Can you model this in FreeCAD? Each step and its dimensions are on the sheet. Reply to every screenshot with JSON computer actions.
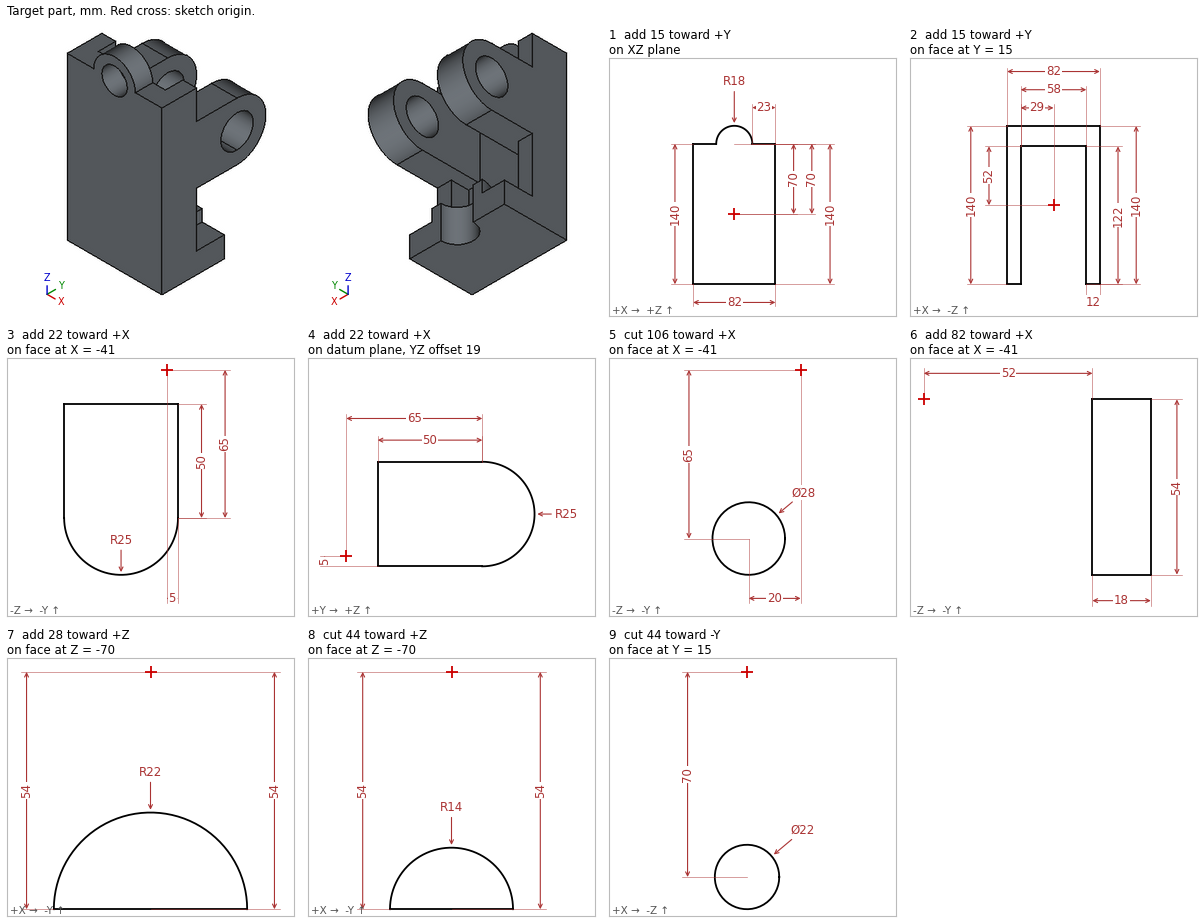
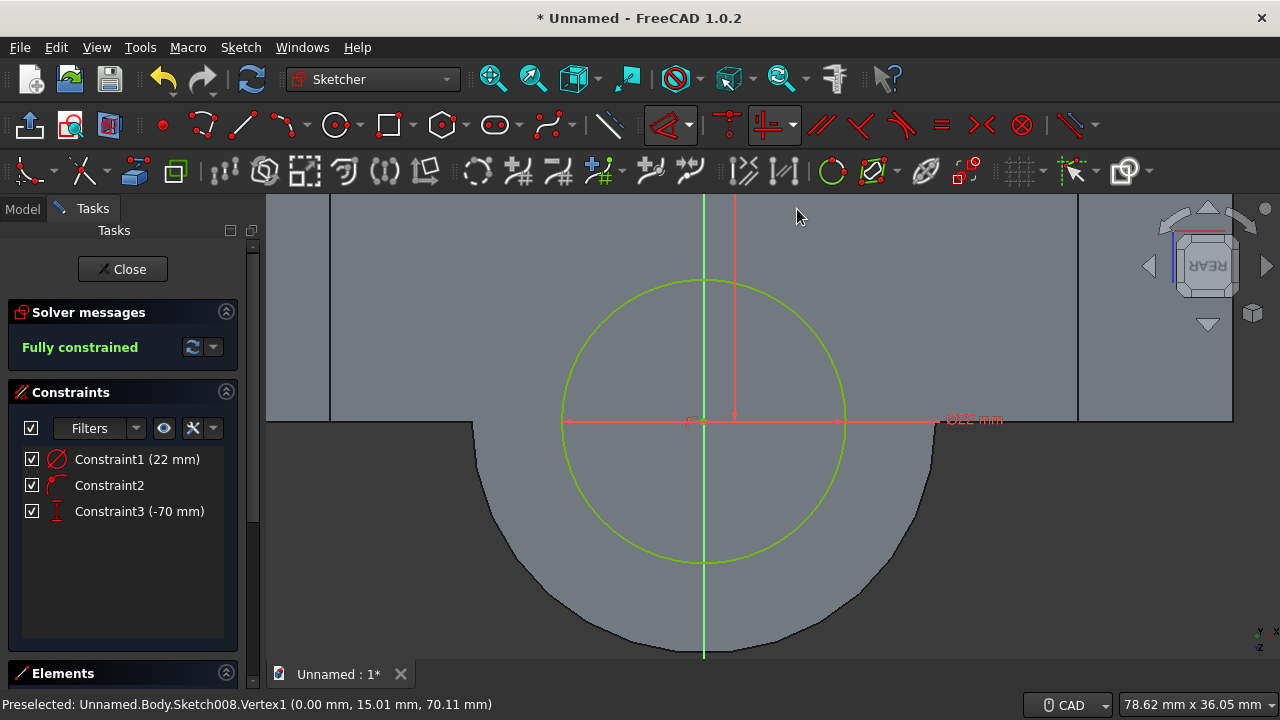
{"action": "left_click", "coordinate": [123, 269]}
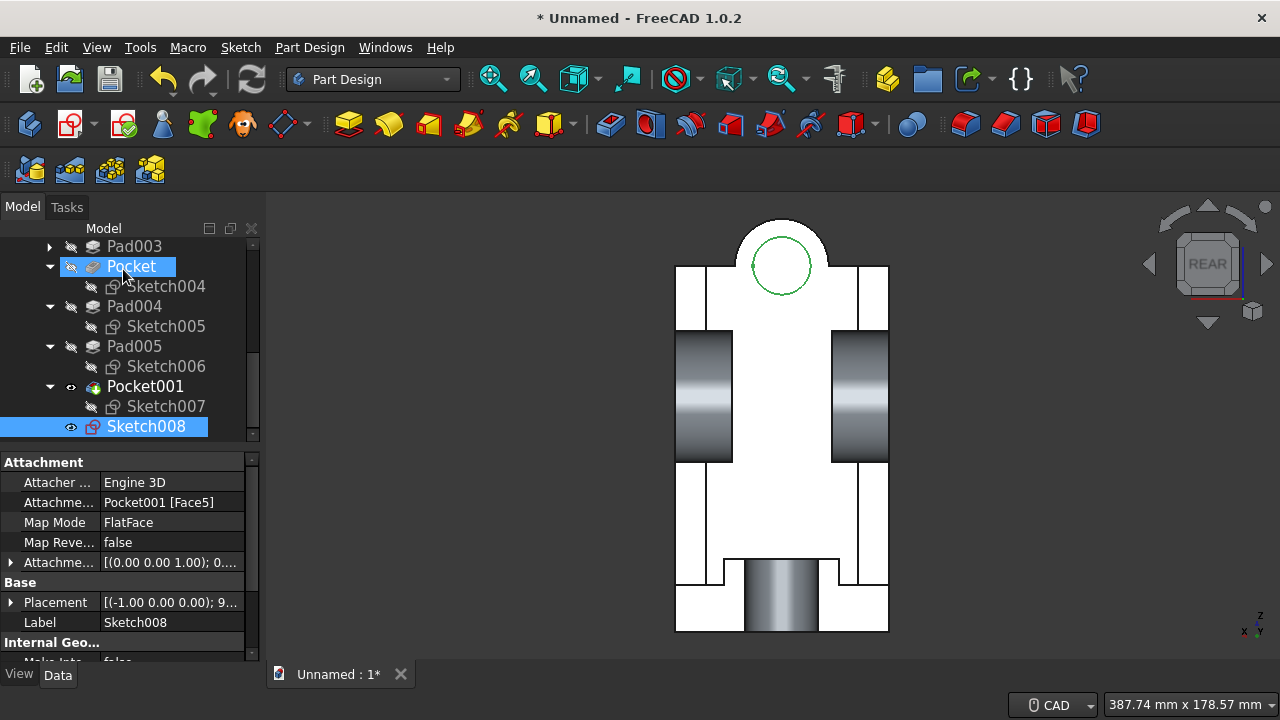
{"action": "left_click", "coordinate": [612, 124]}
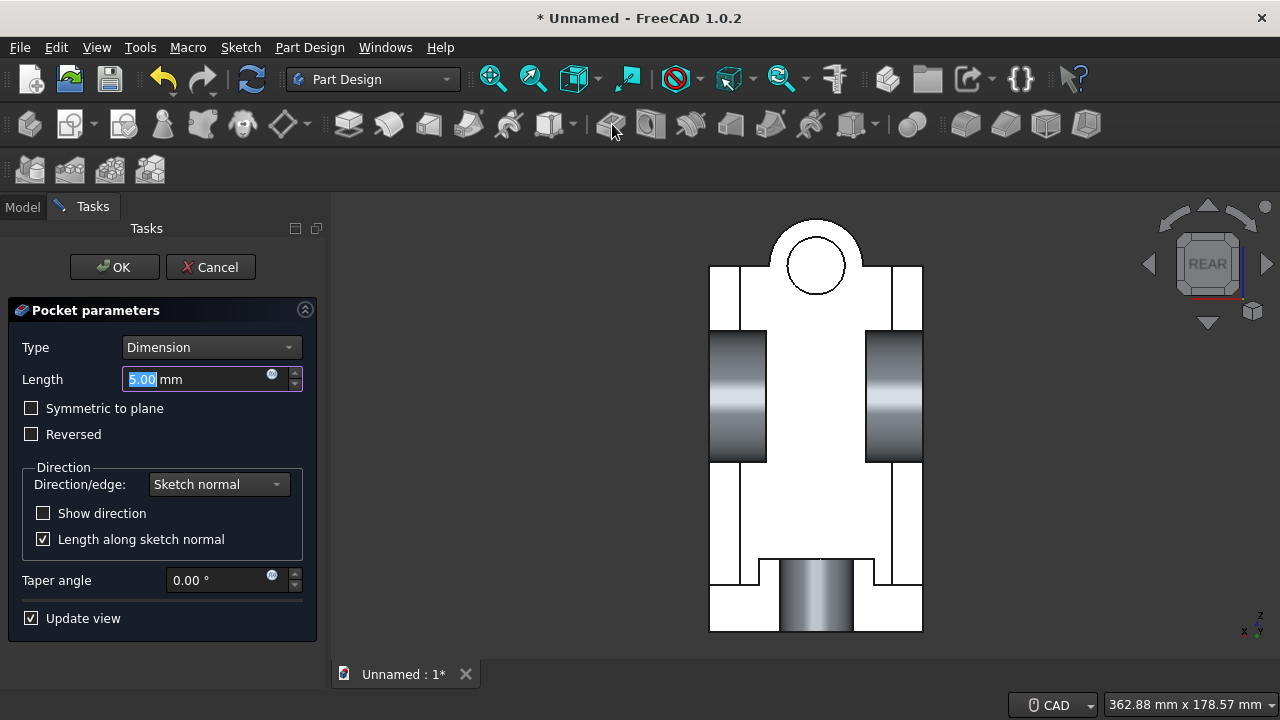
{"action": "type", "text": "44"}
{"action": "key", "text": "Tab"}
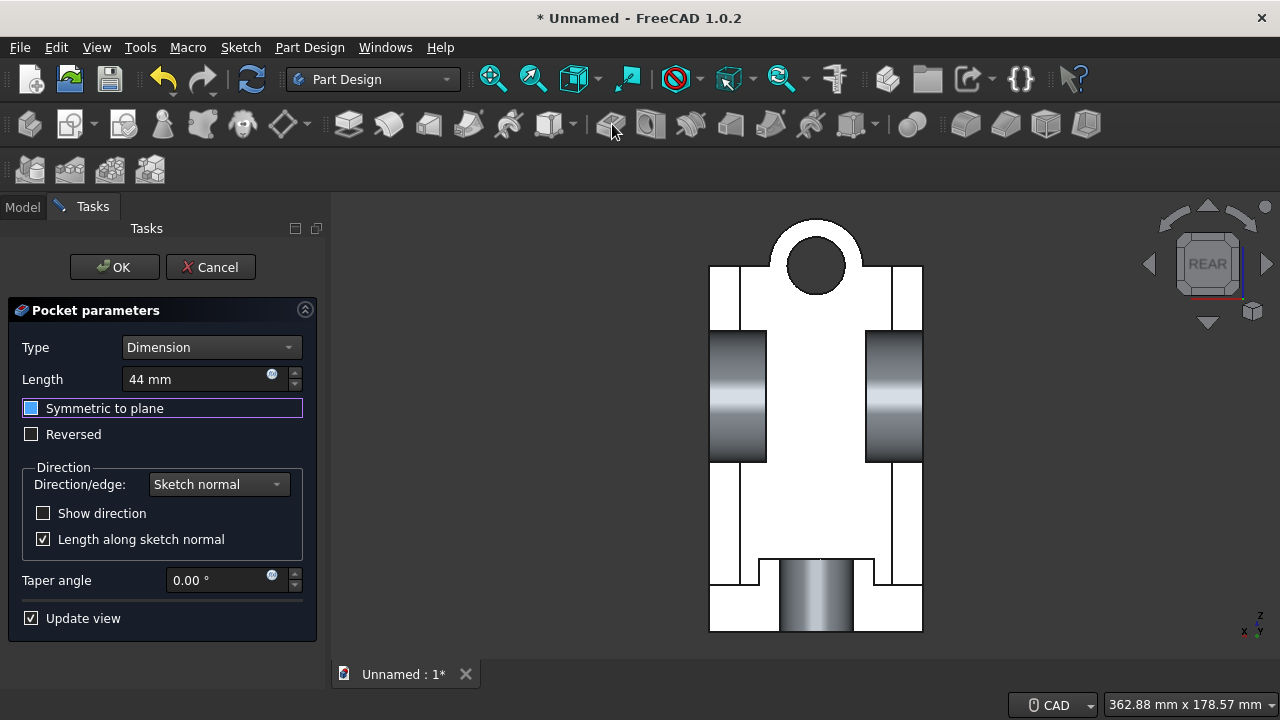
{"action": "left_click", "coordinate": [115, 267]}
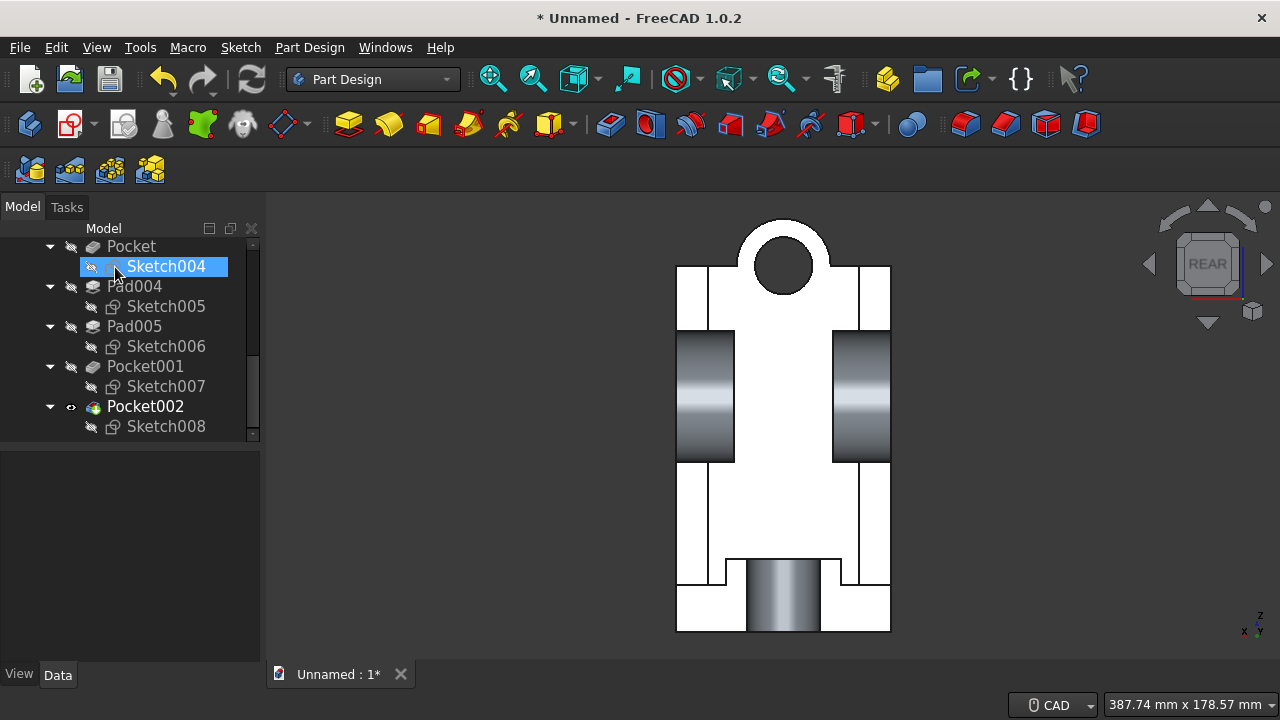
{"action": "key", "text": "0"}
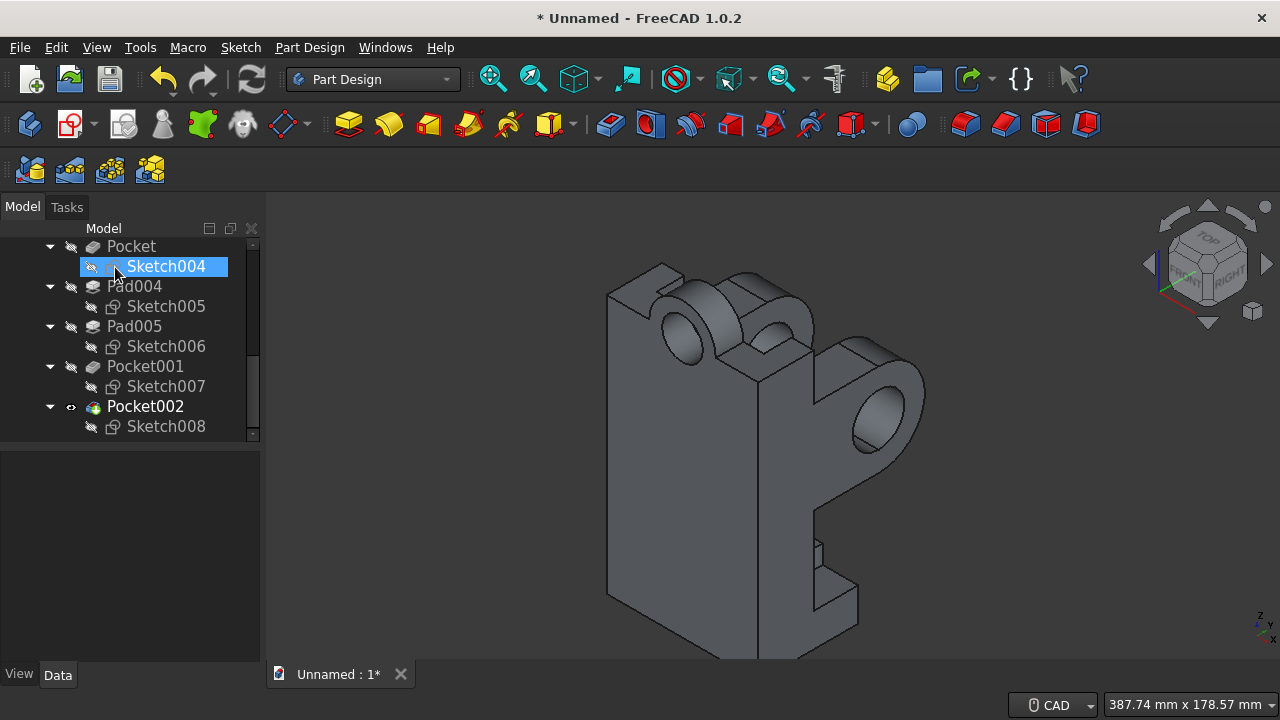
{"action": "key", "text": "v f"}